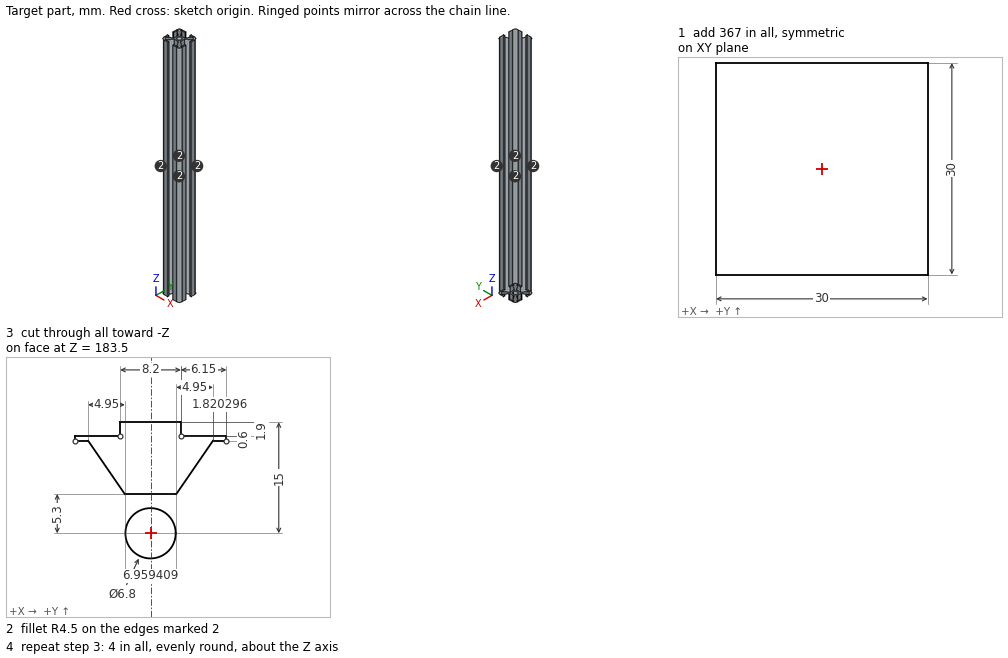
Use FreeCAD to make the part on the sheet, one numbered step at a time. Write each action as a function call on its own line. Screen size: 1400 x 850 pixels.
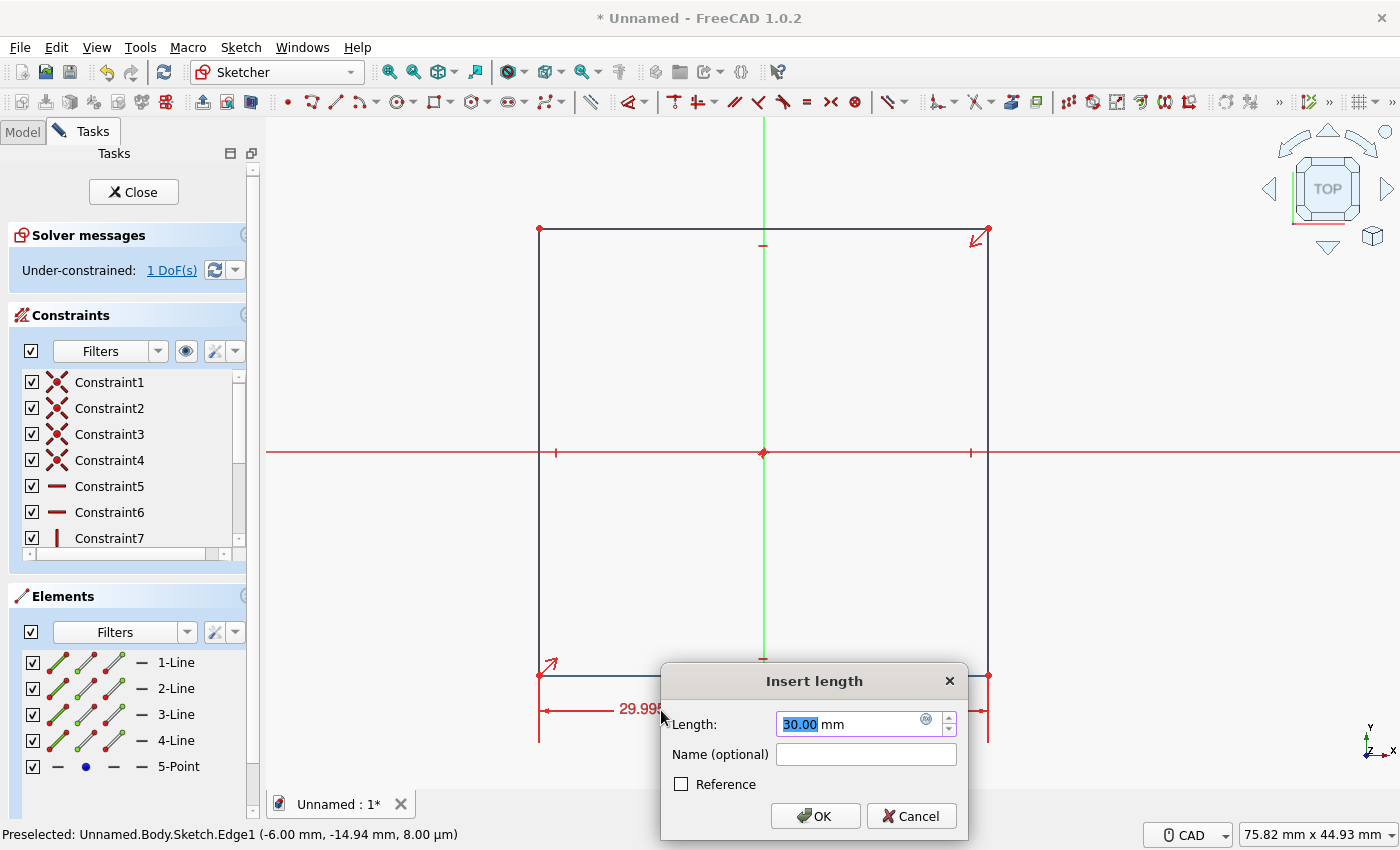
text(30)
key(Return)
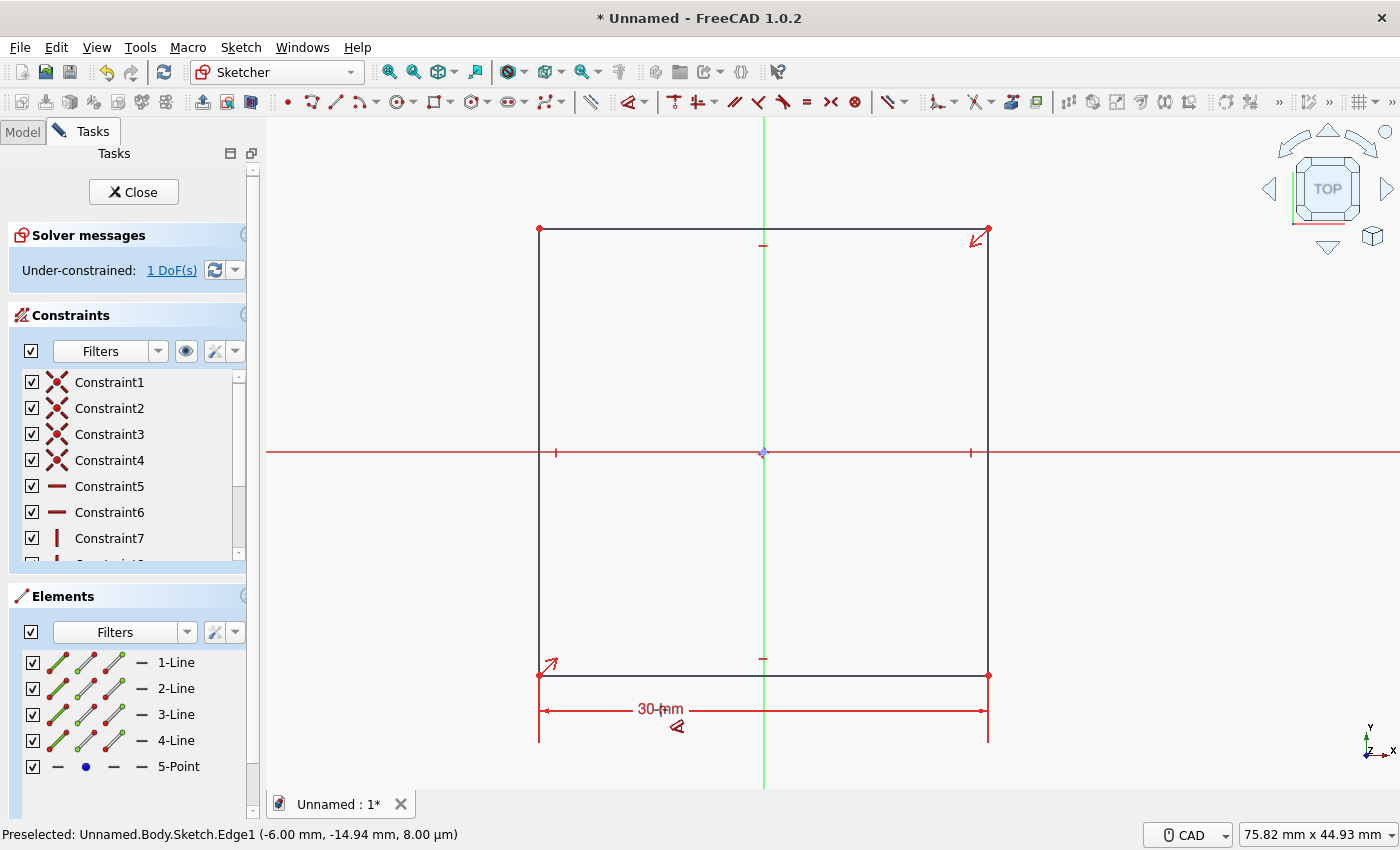
click(988, 542)
click(1022, 350)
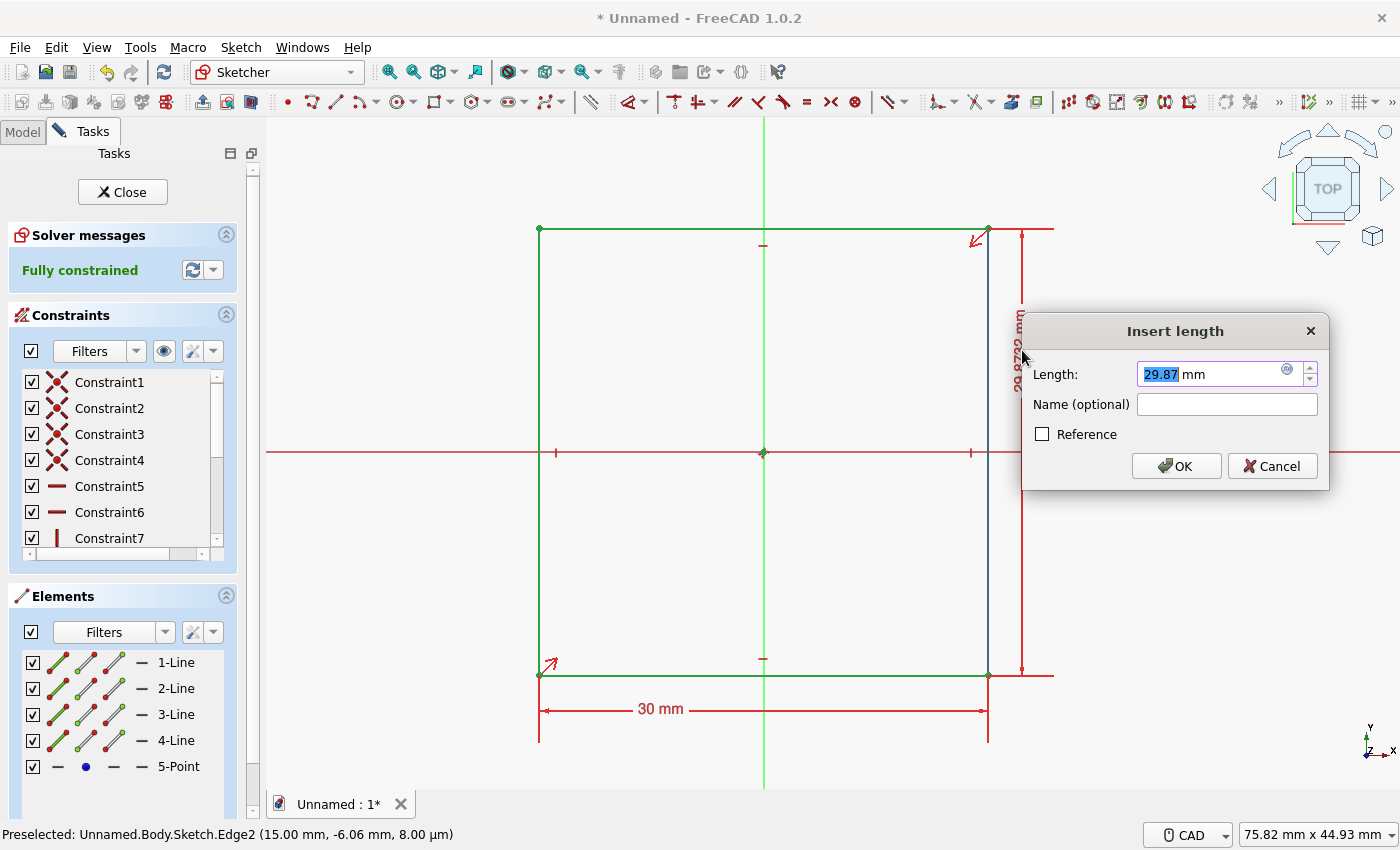
text(30)
key(Return)
key(Escape)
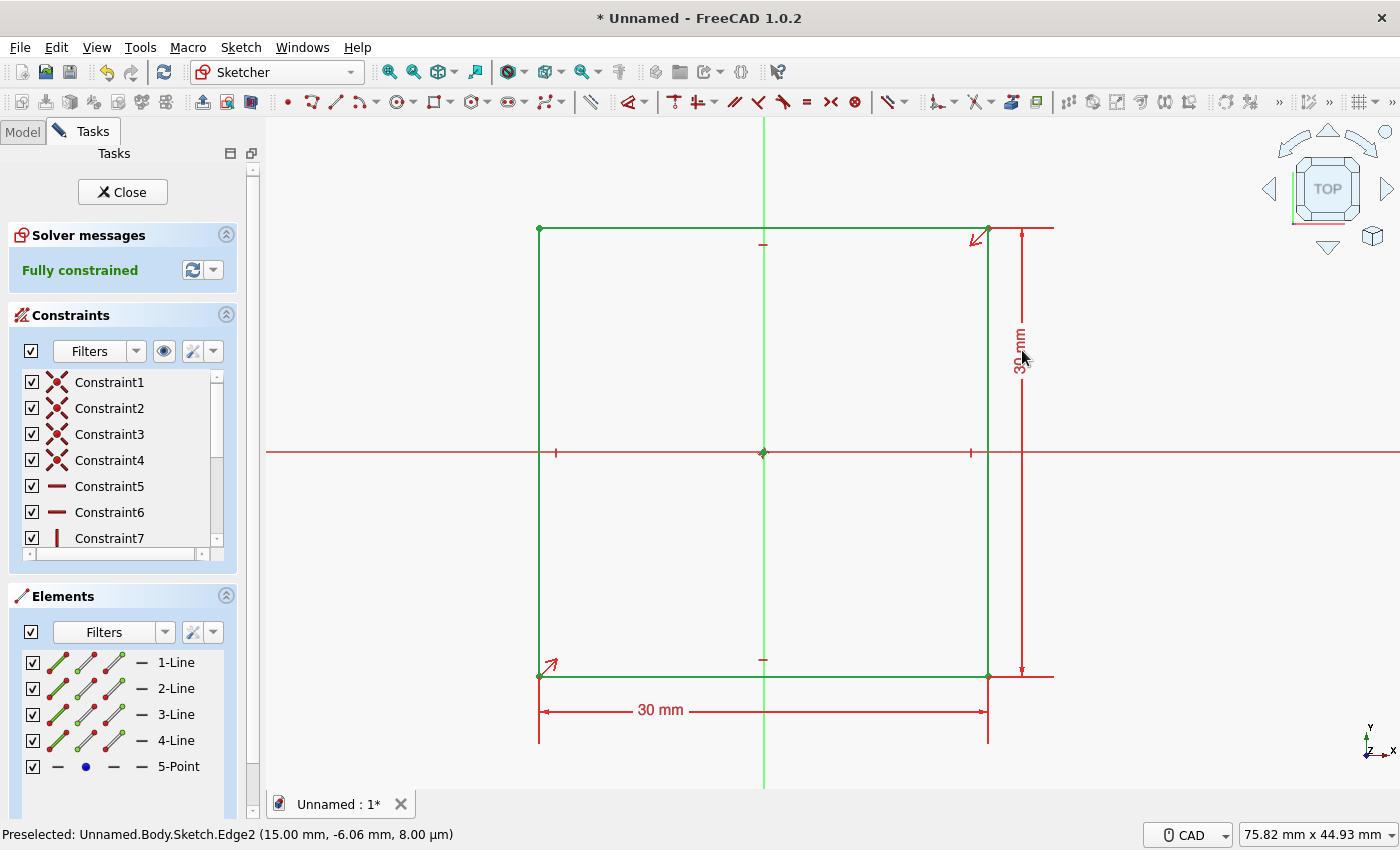
click(123, 192)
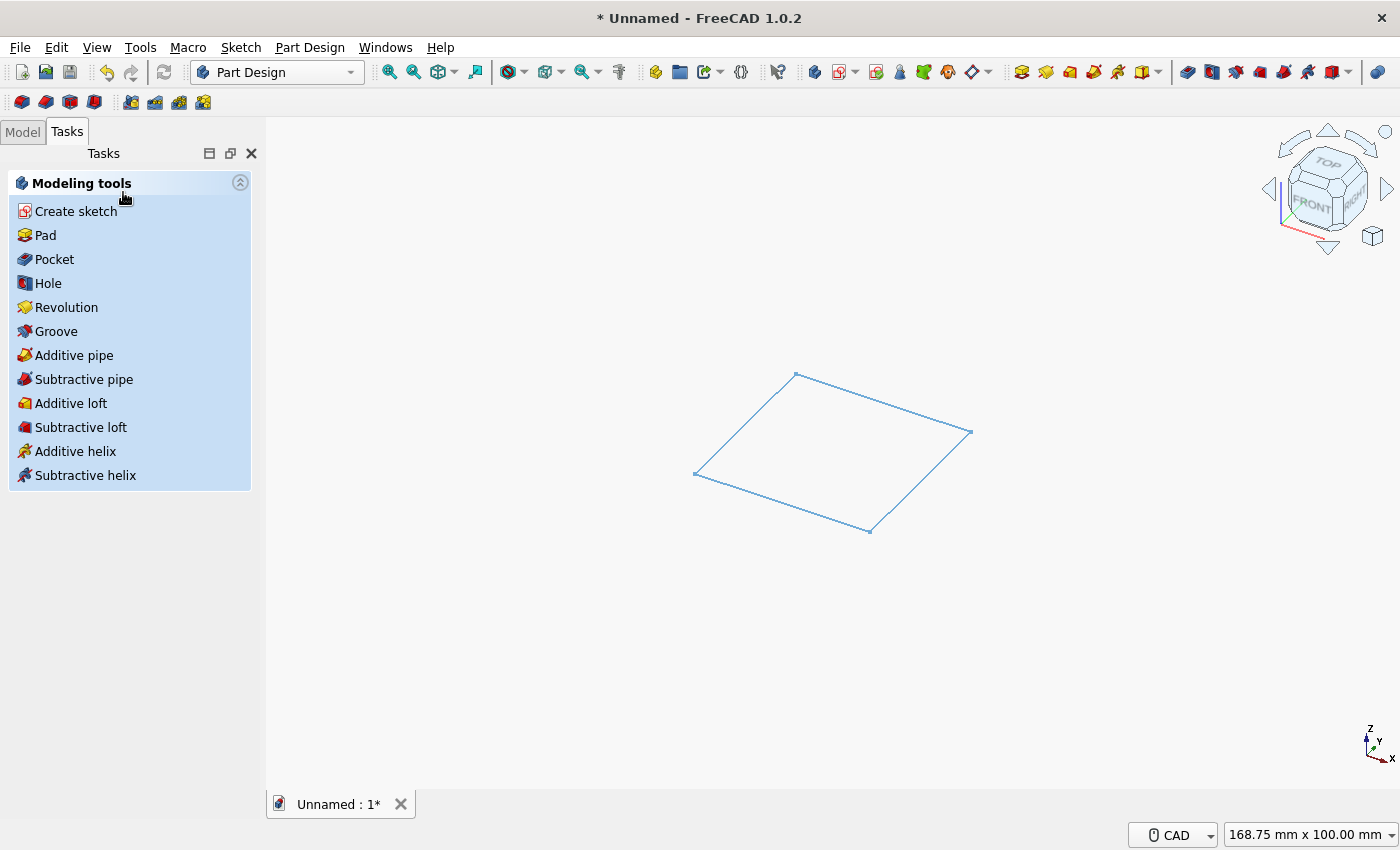
click(1022, 72)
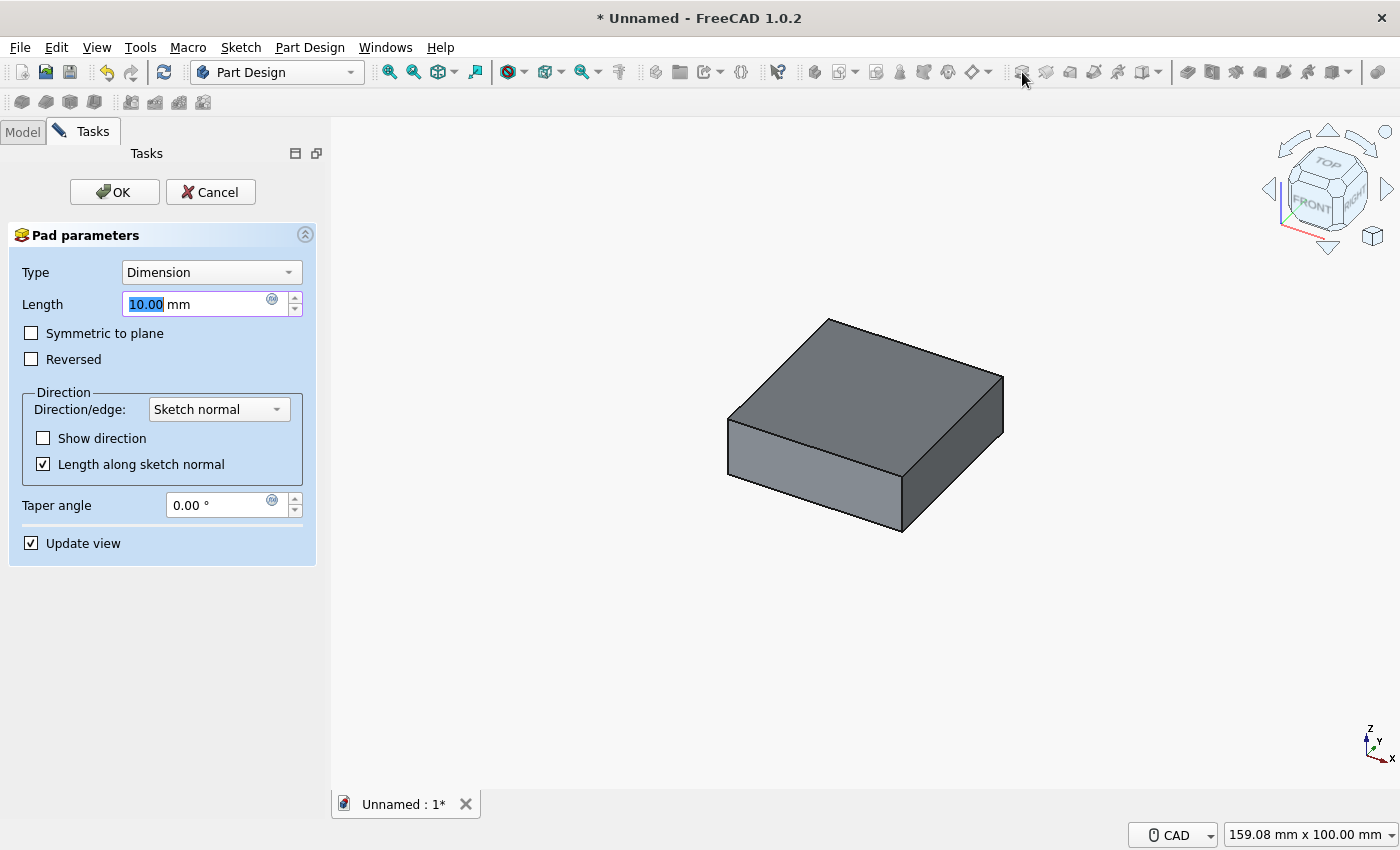
text(367)
key(Tab)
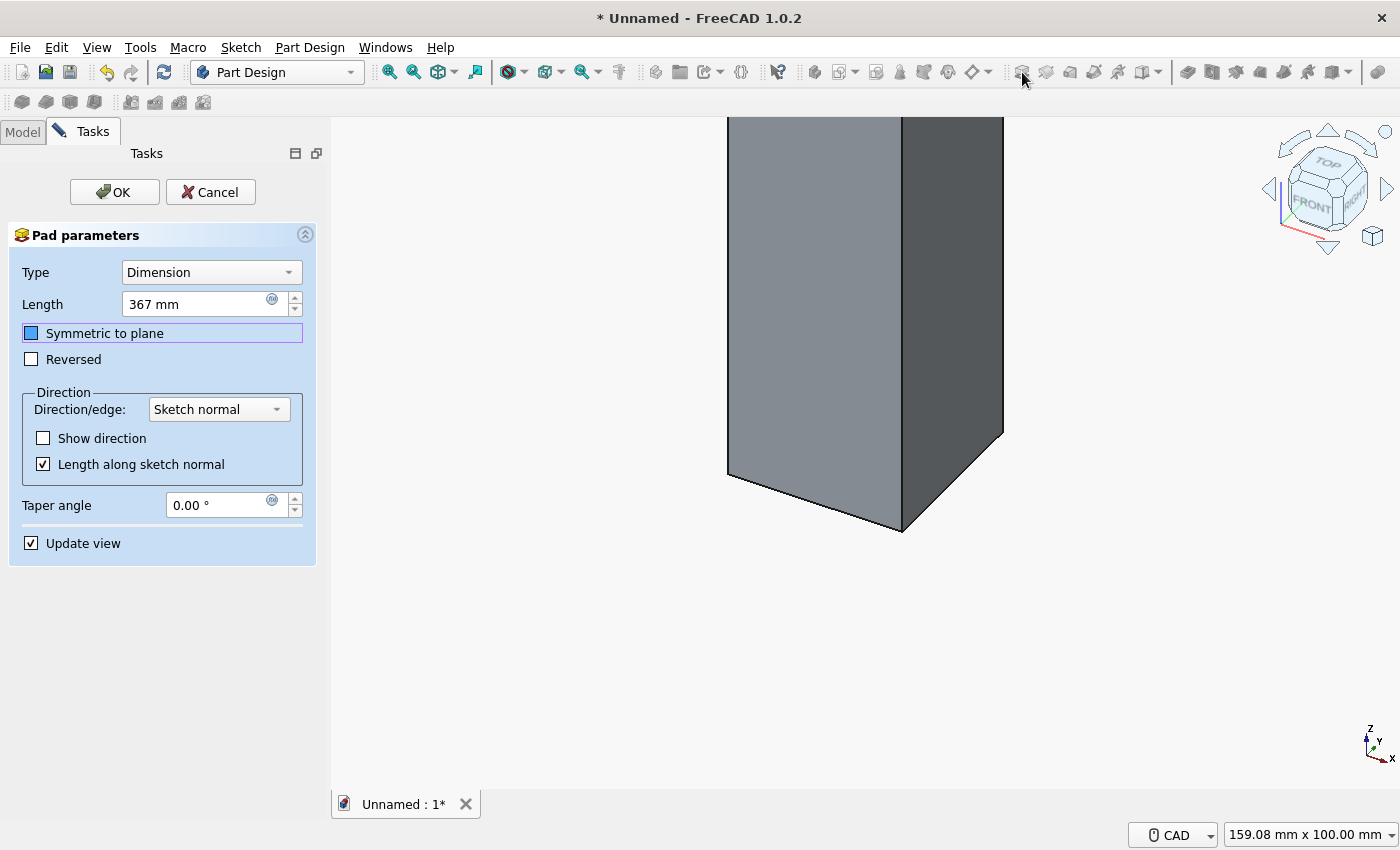
click(30, 333)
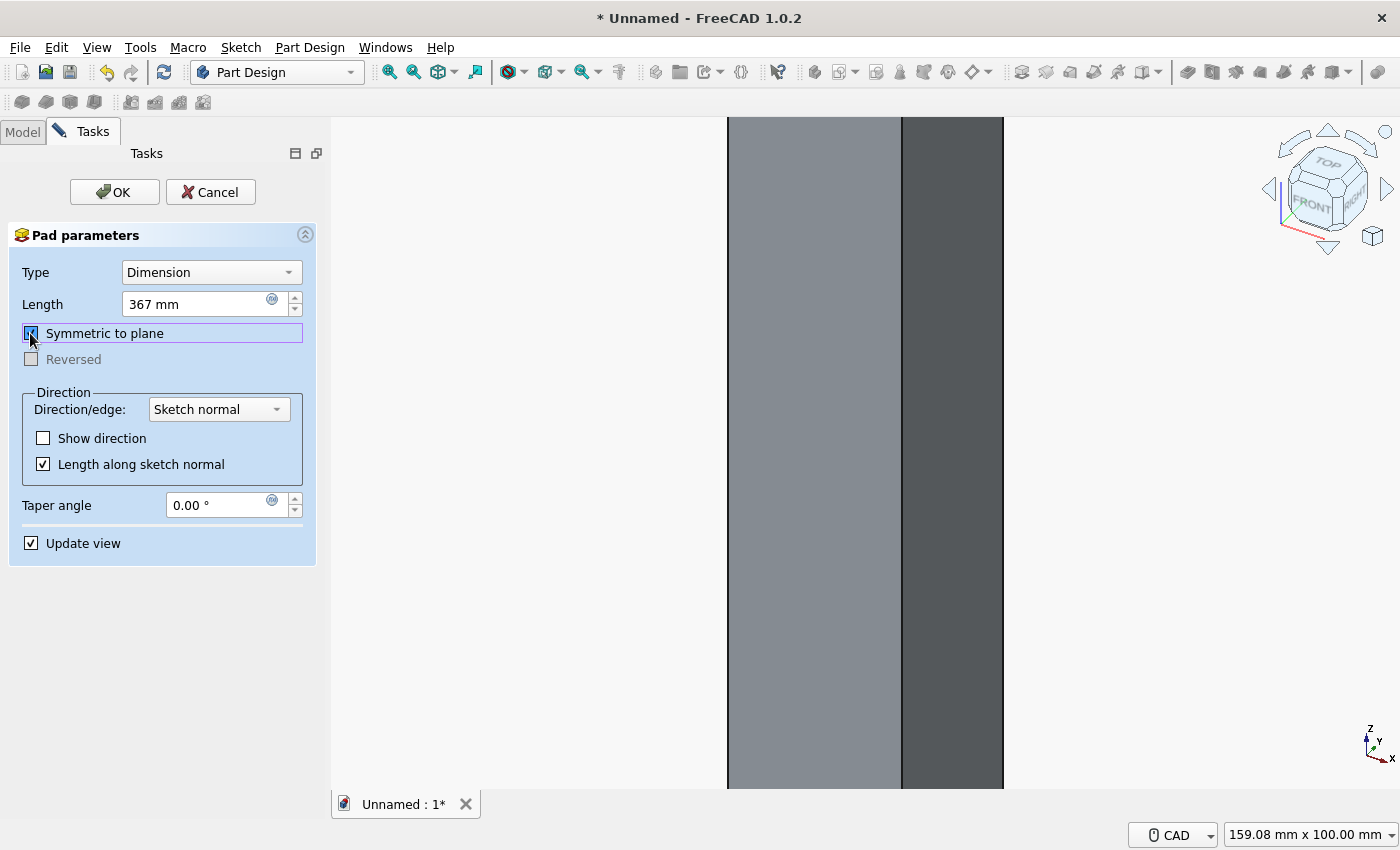
click(115, 192)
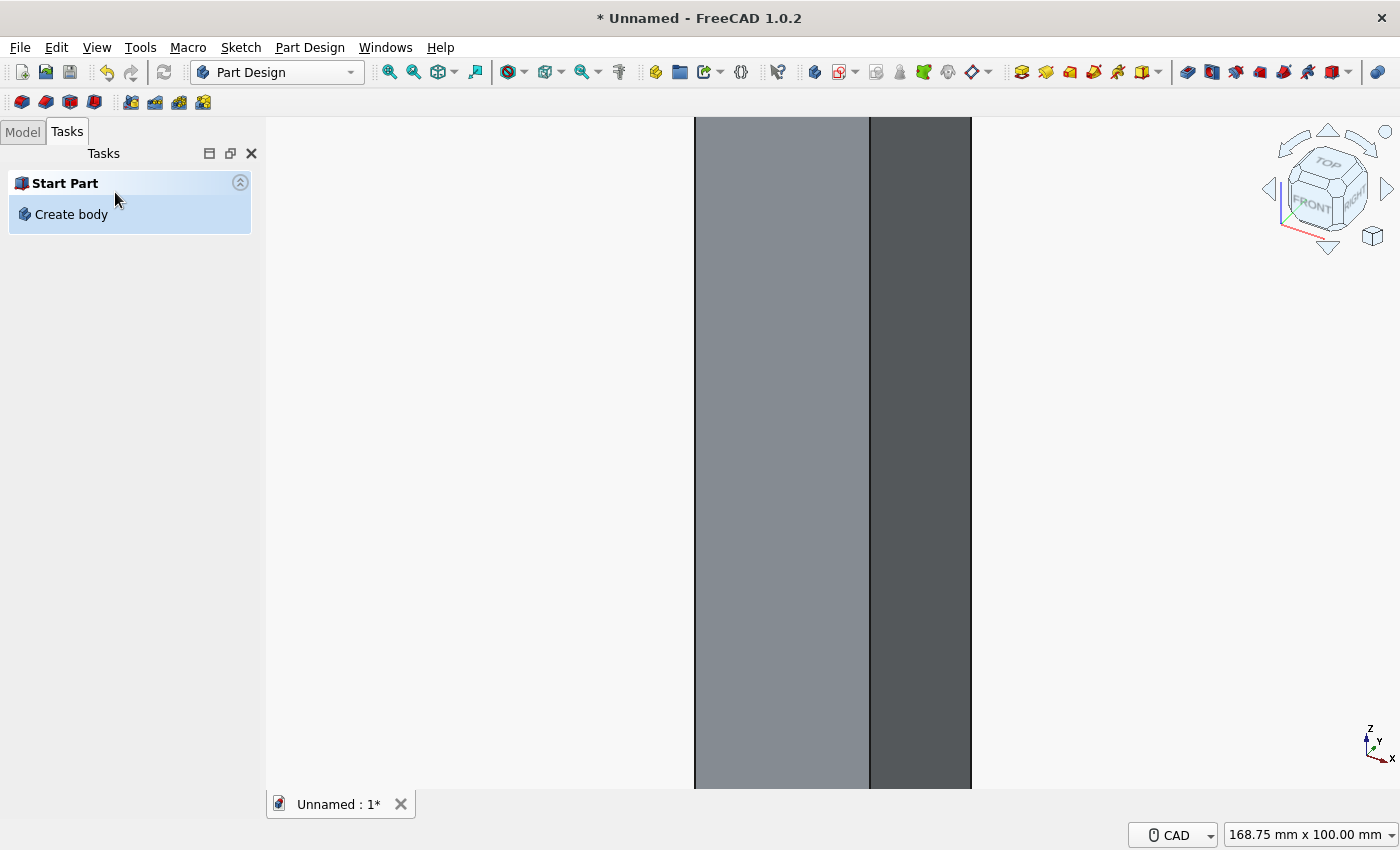
key(v)
key(f)